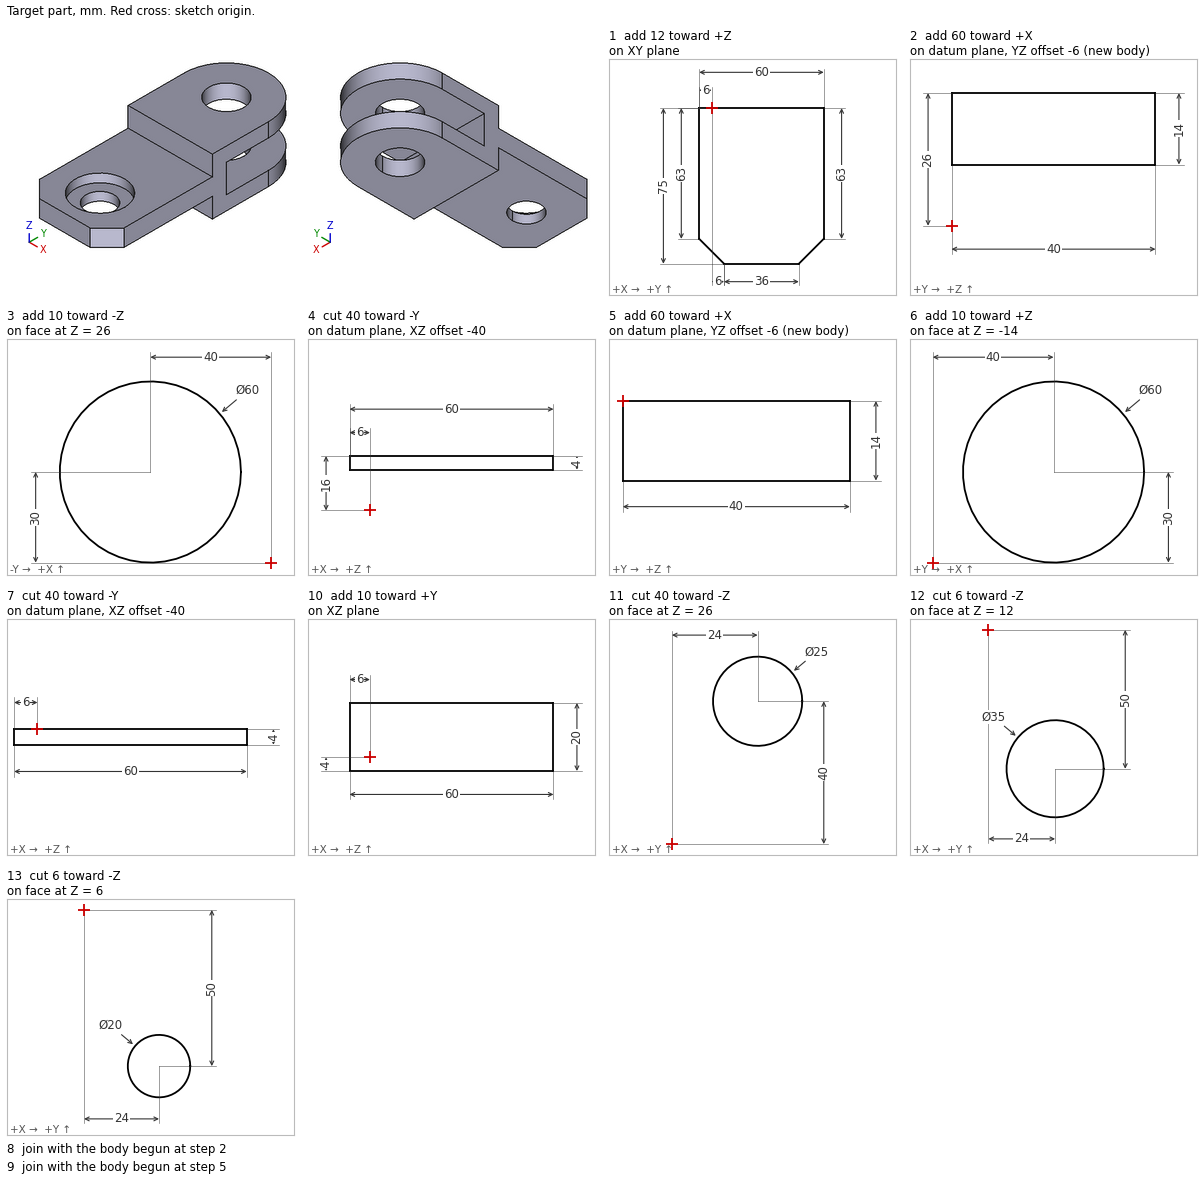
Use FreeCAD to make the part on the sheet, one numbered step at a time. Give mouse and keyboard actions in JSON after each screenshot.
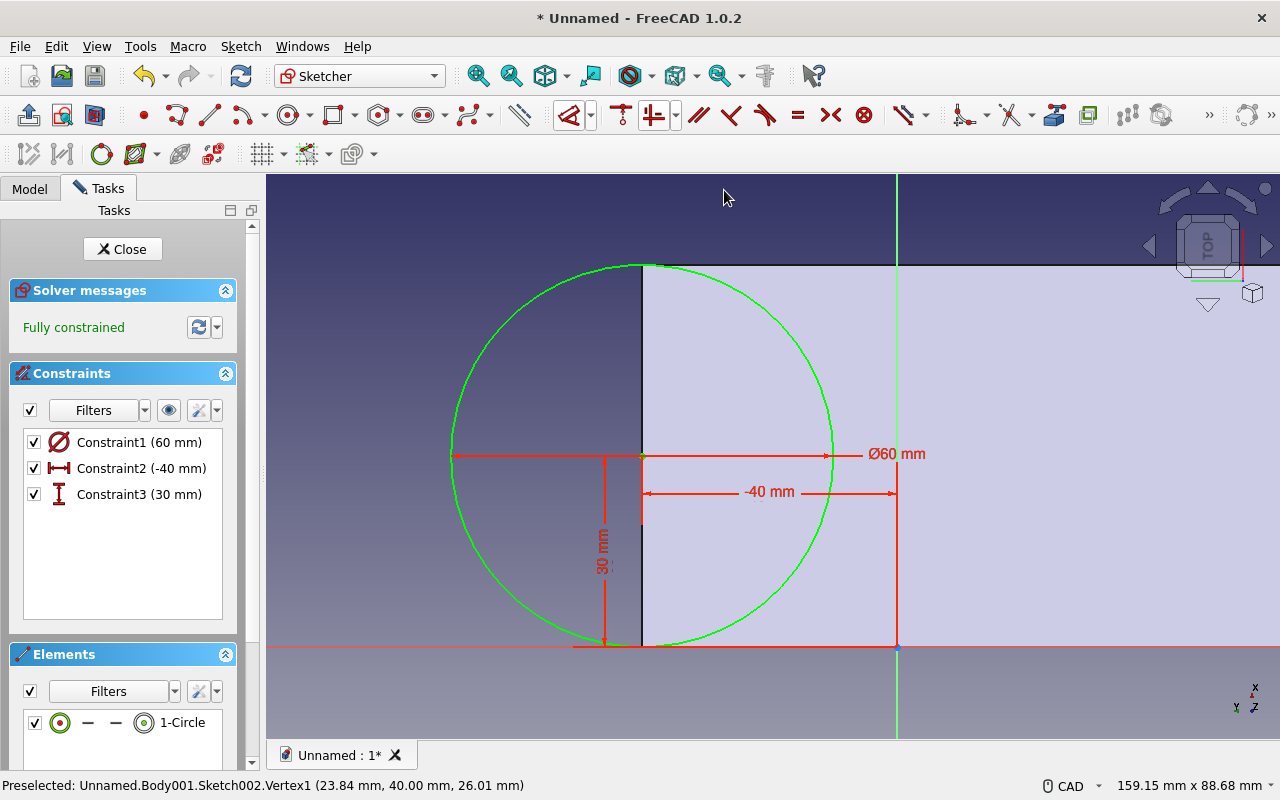
{"action": "left_click", "coordinate": [123, 249]}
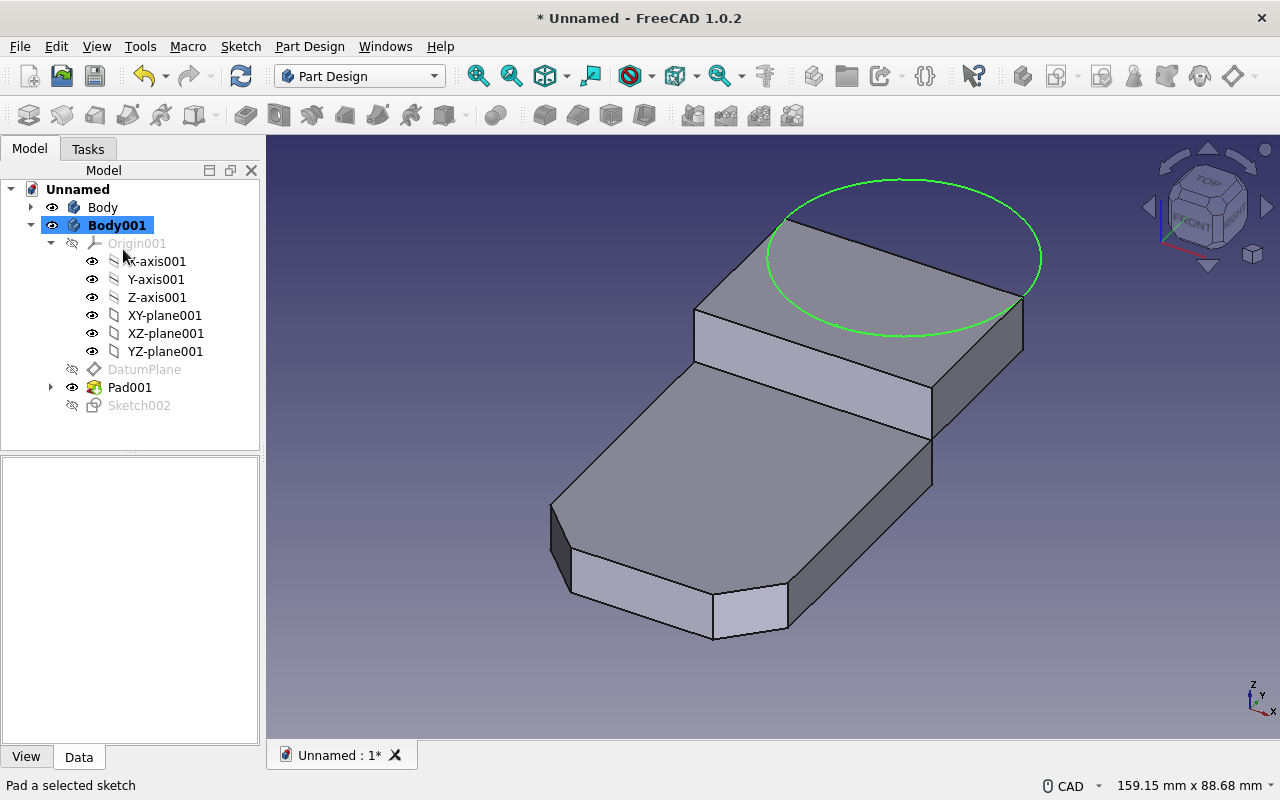
{"action": "left_click", "coordinate": [29, 116]}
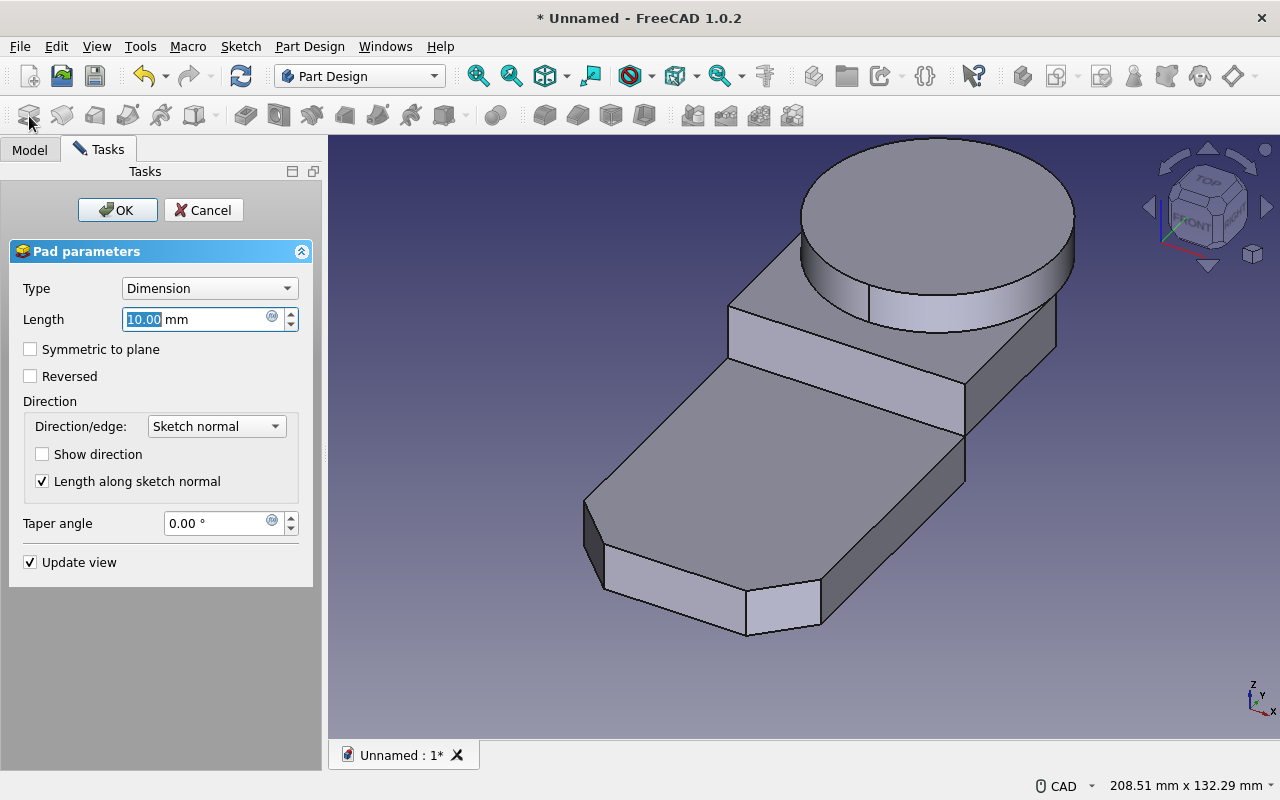
{"action": "type", "text": "10"}
{"action": "key", "text": "Tab"}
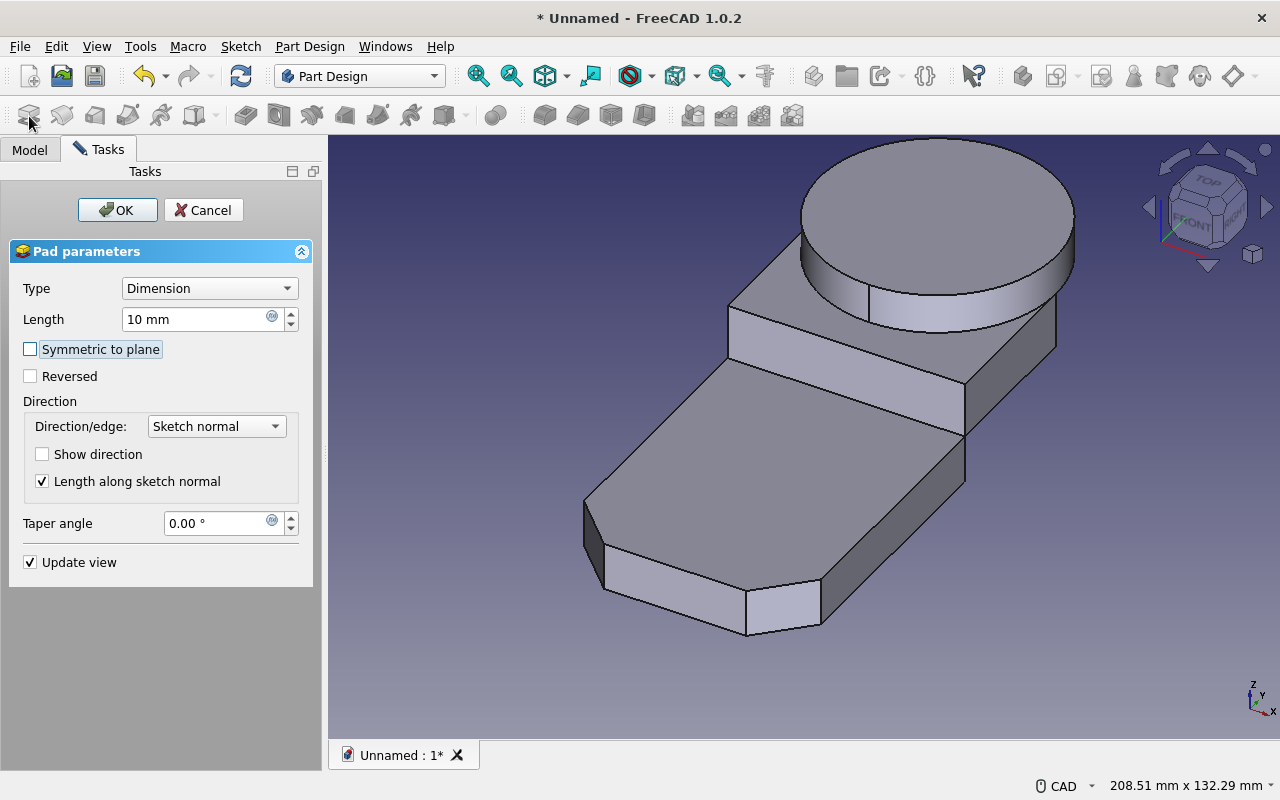
{"action": "left_click", "coordinate": [31, 376]}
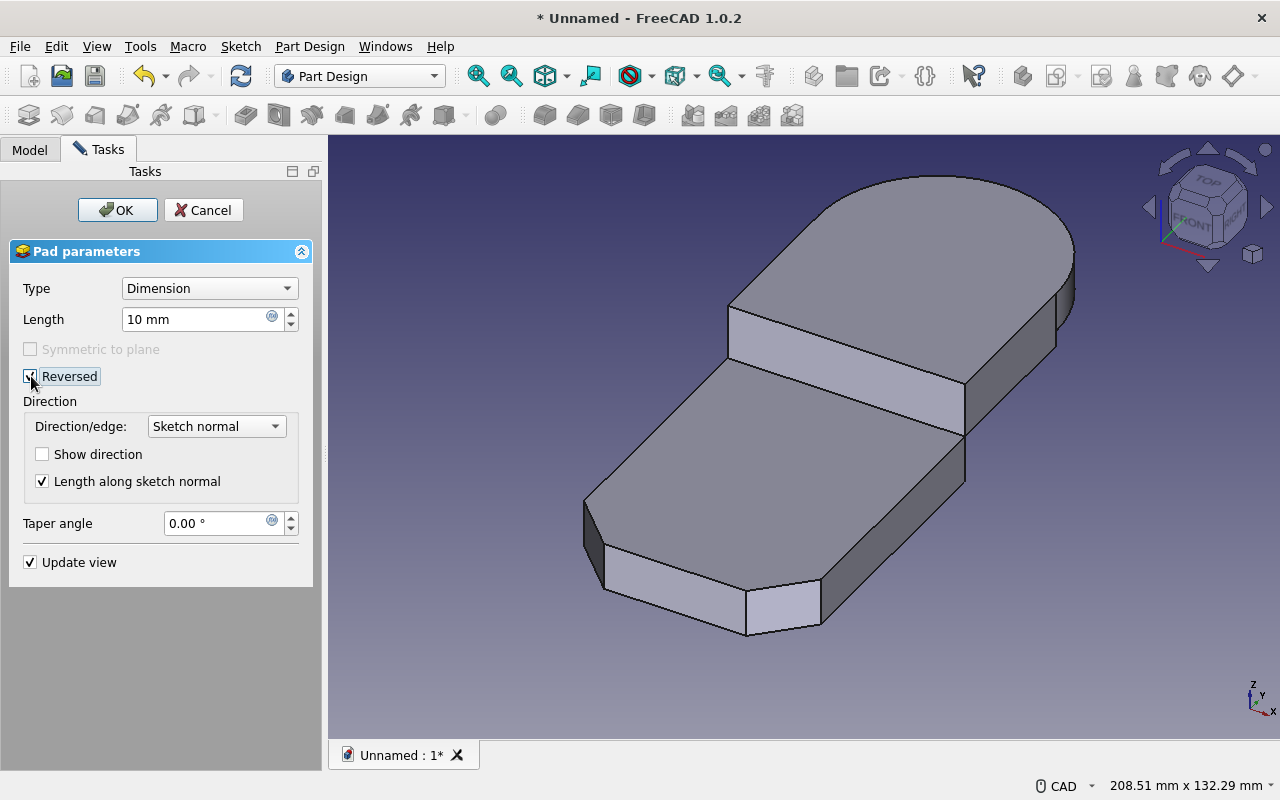
{"action": "left_click", "coordinate": [118, 210]}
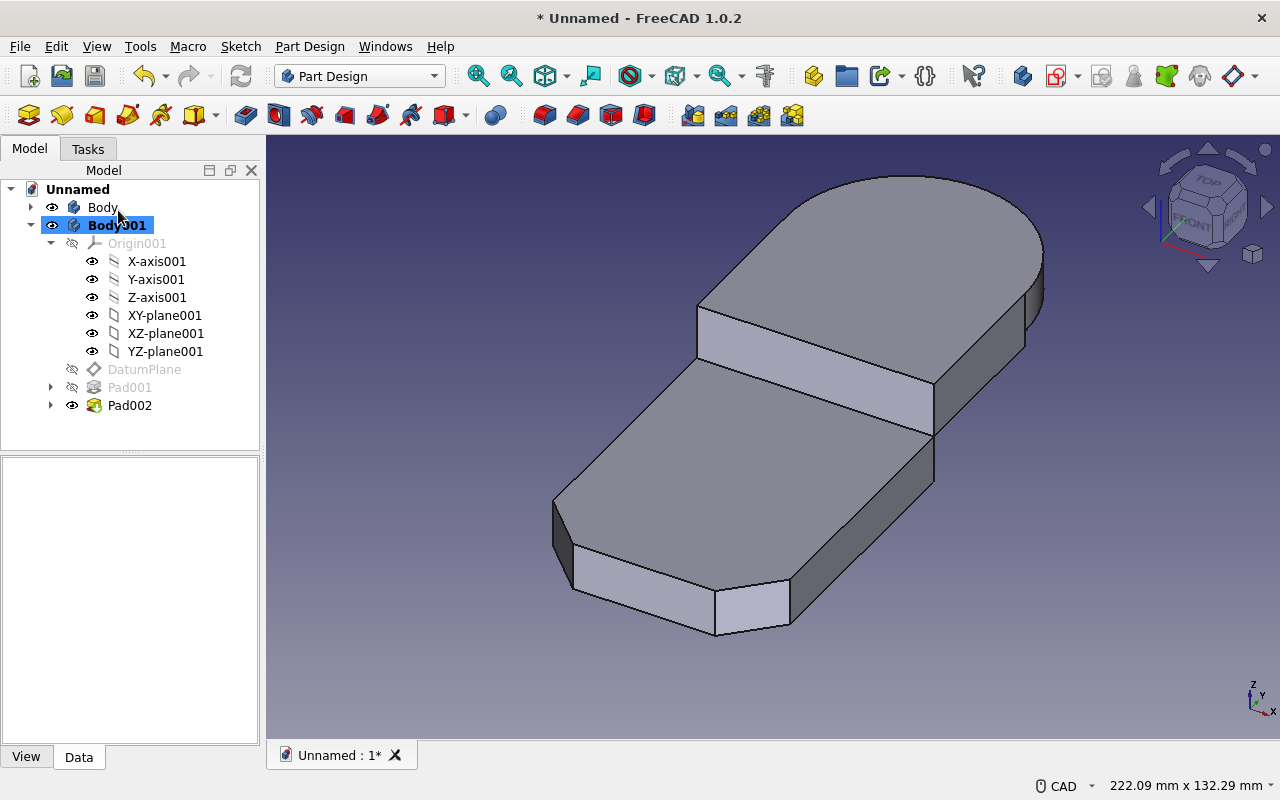
{"action": "key", "text": "4"}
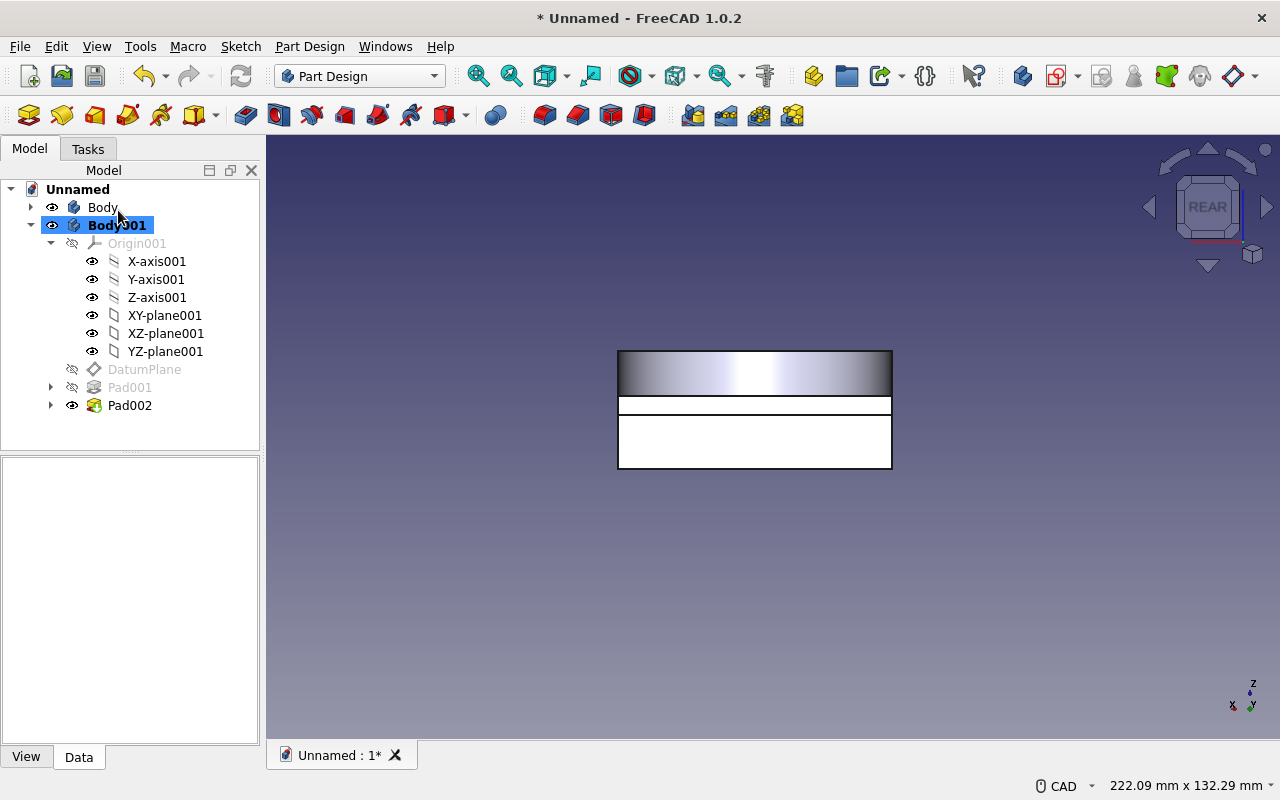
{"action": "key", "text": "v f"}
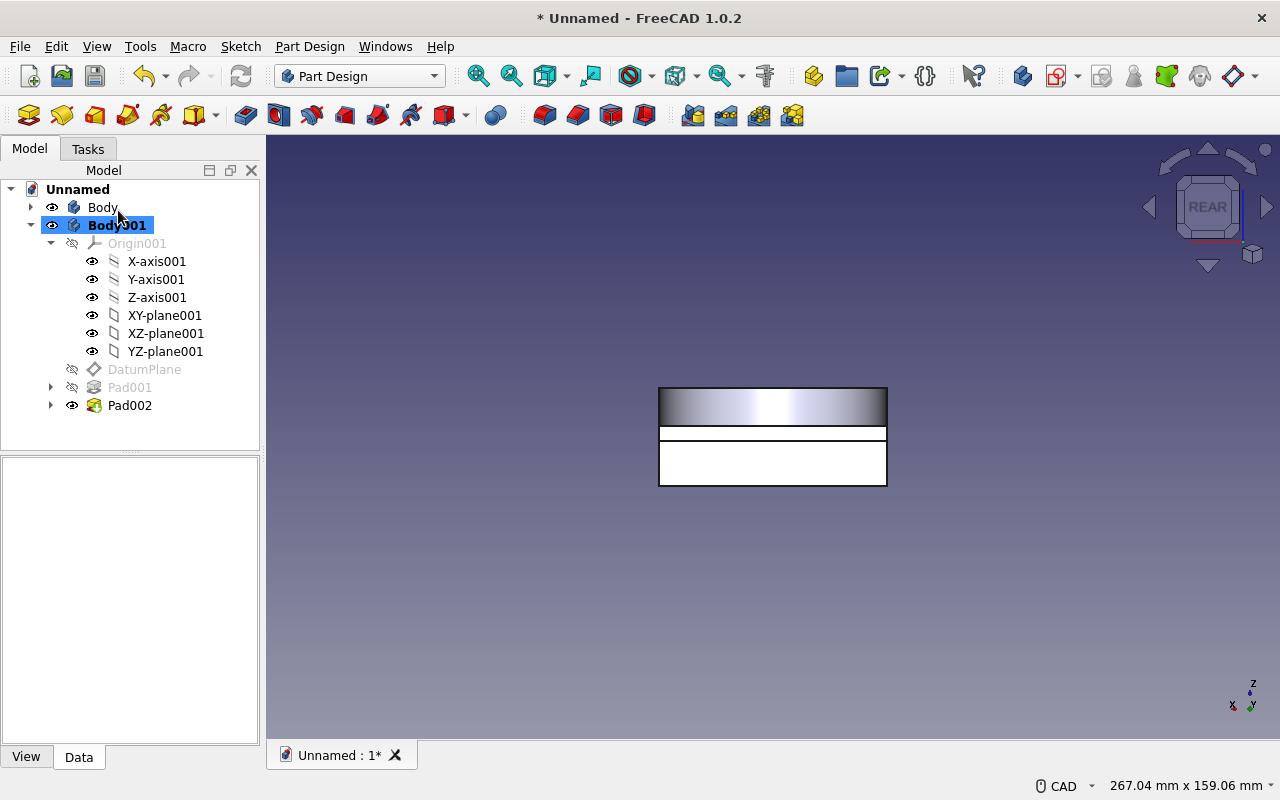
{"action": "key", "text": "5"}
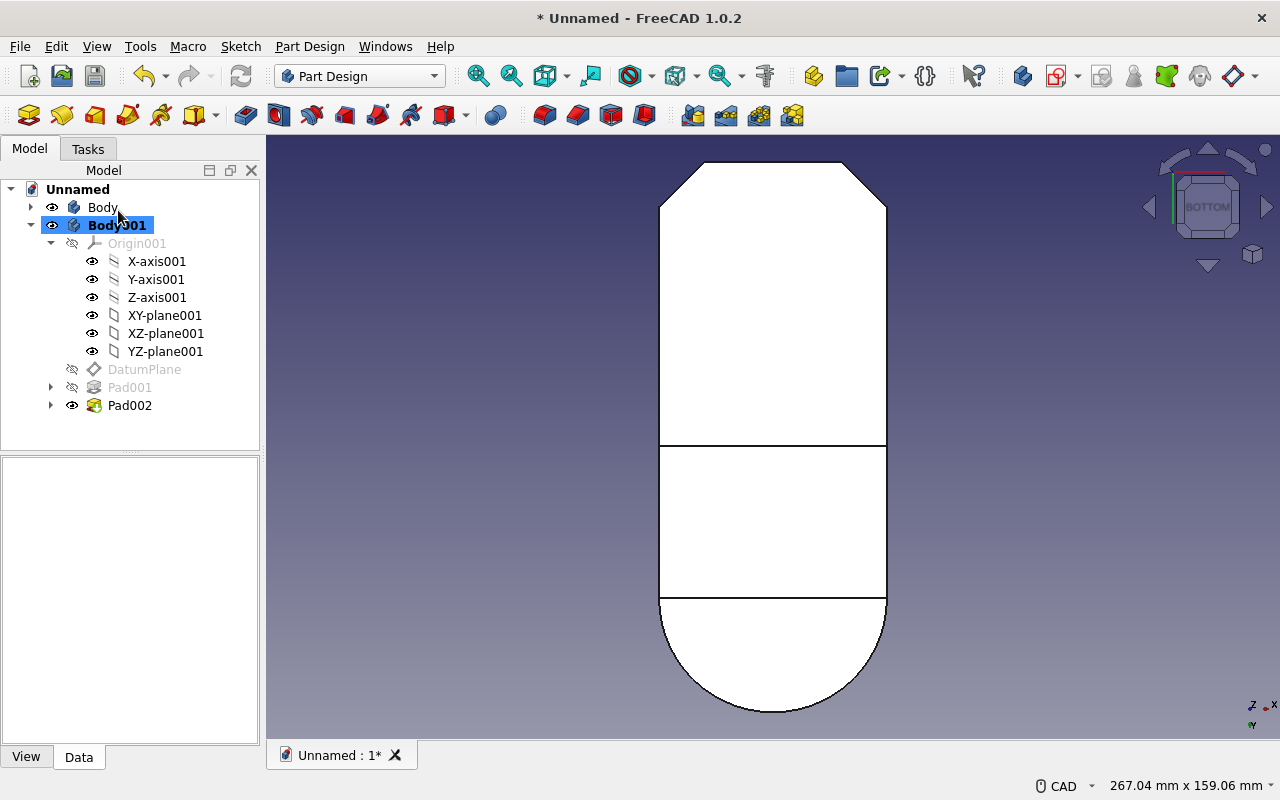
{"action": "left_click", "coordinate": [479, 76]}